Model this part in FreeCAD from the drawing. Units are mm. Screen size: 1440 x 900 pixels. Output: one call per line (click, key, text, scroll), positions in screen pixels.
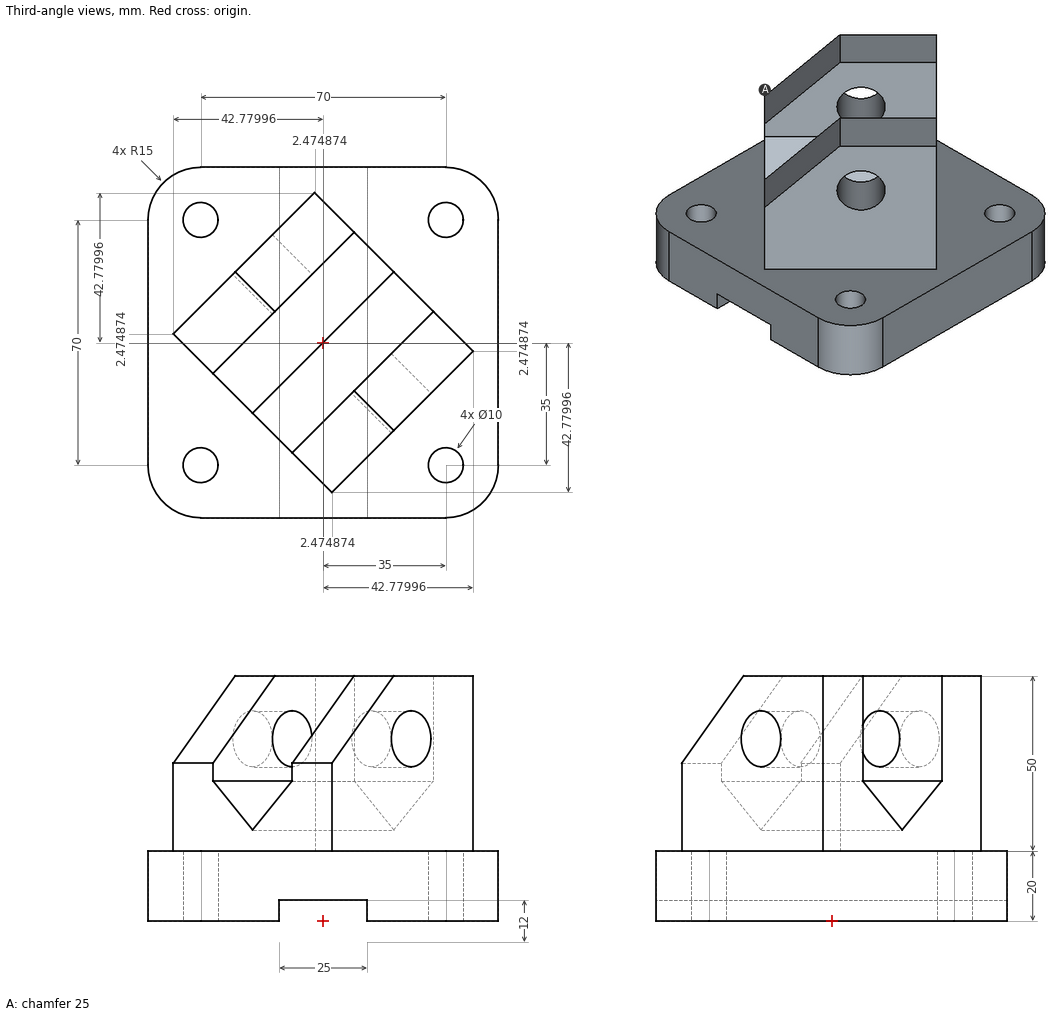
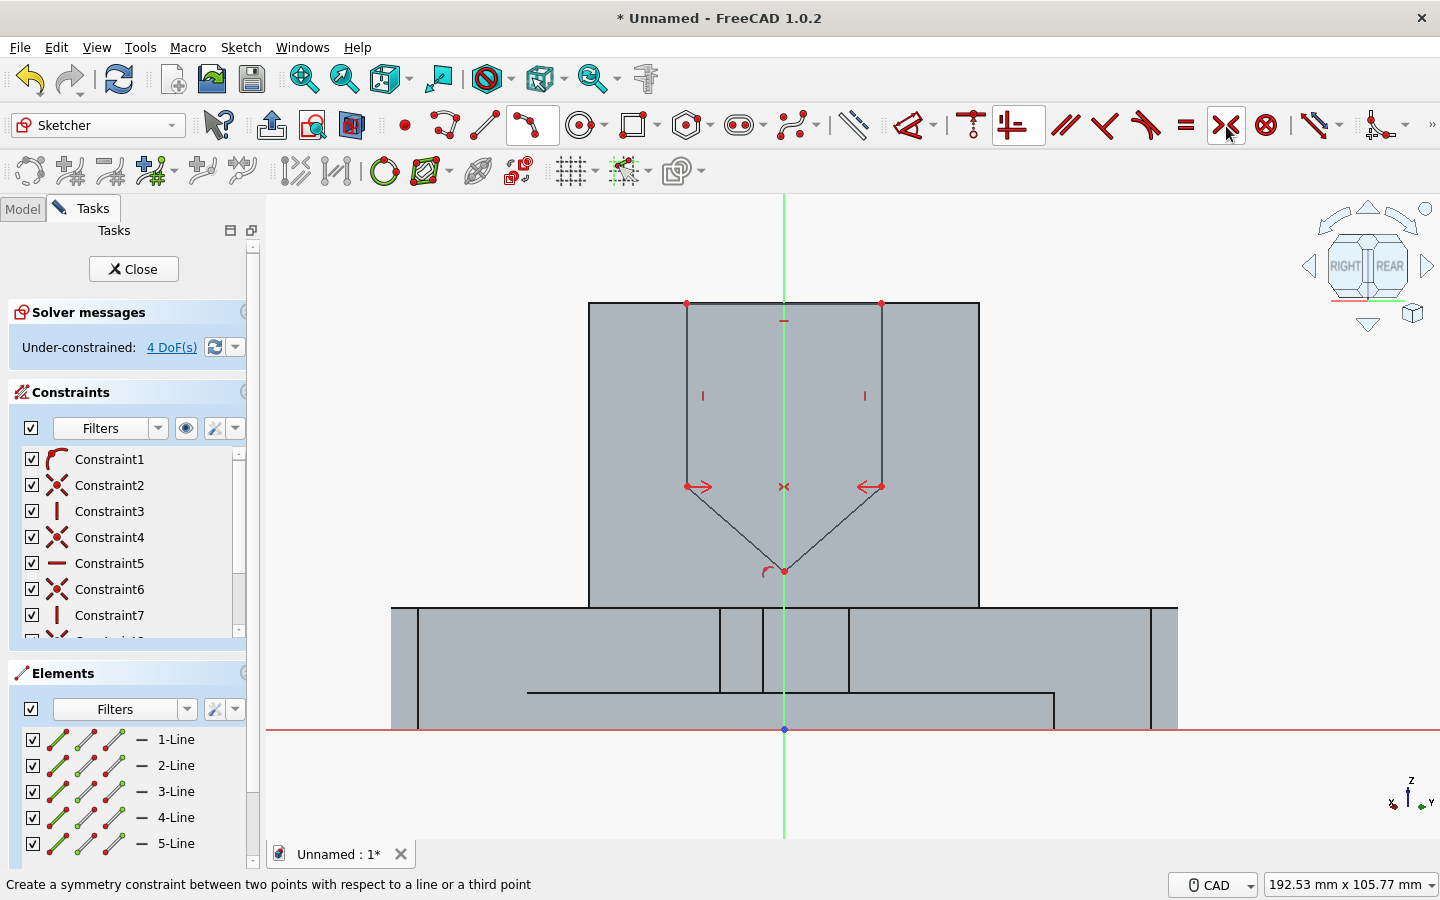
key(d)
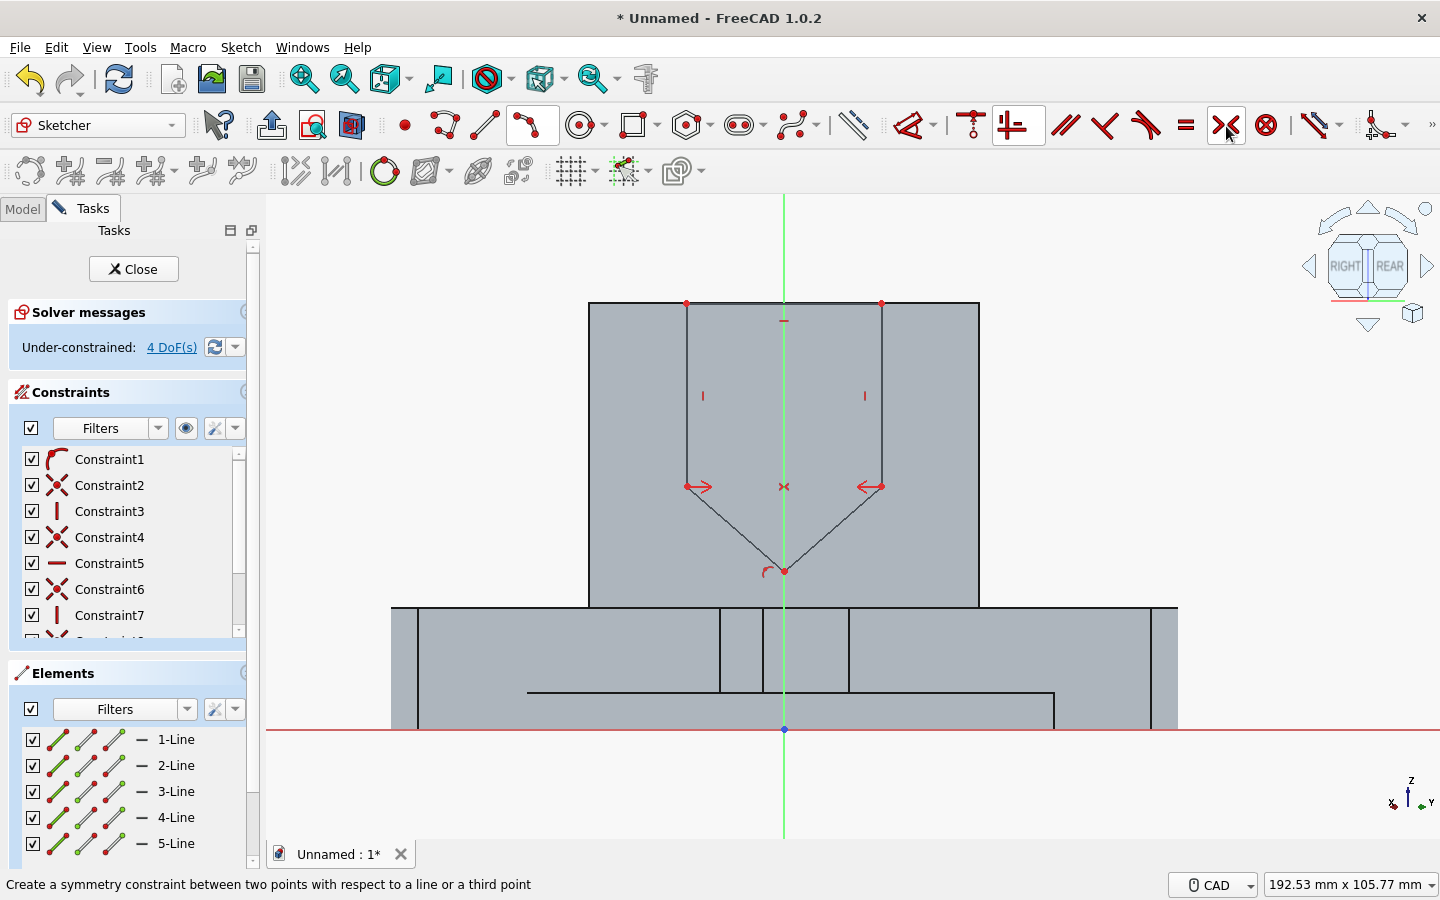
click(882, 432)
click(916, 396)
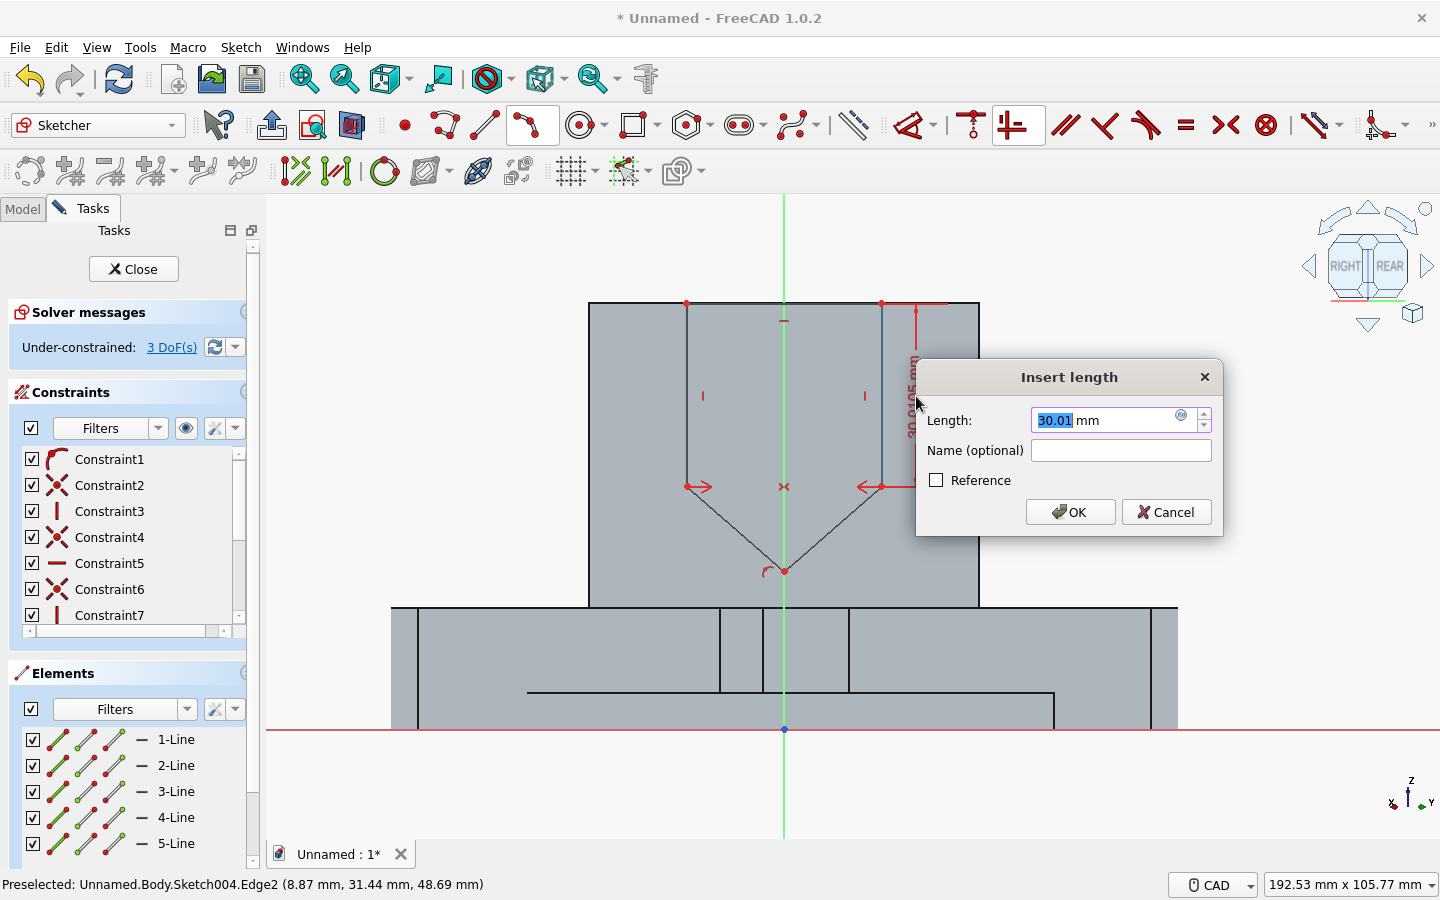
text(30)
key(Return)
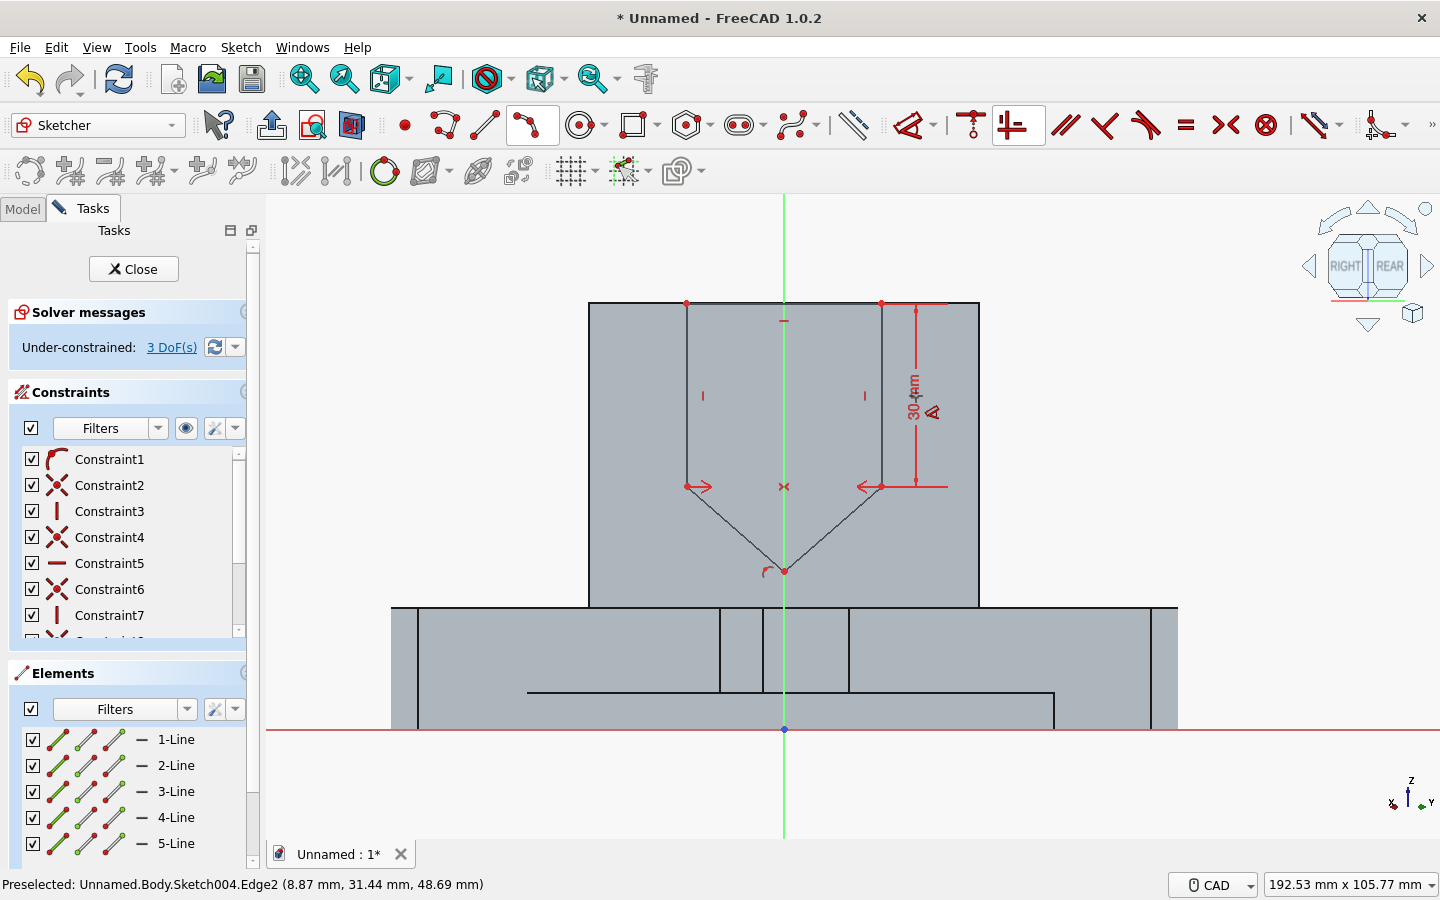
click(823, 304)
click(740, 270)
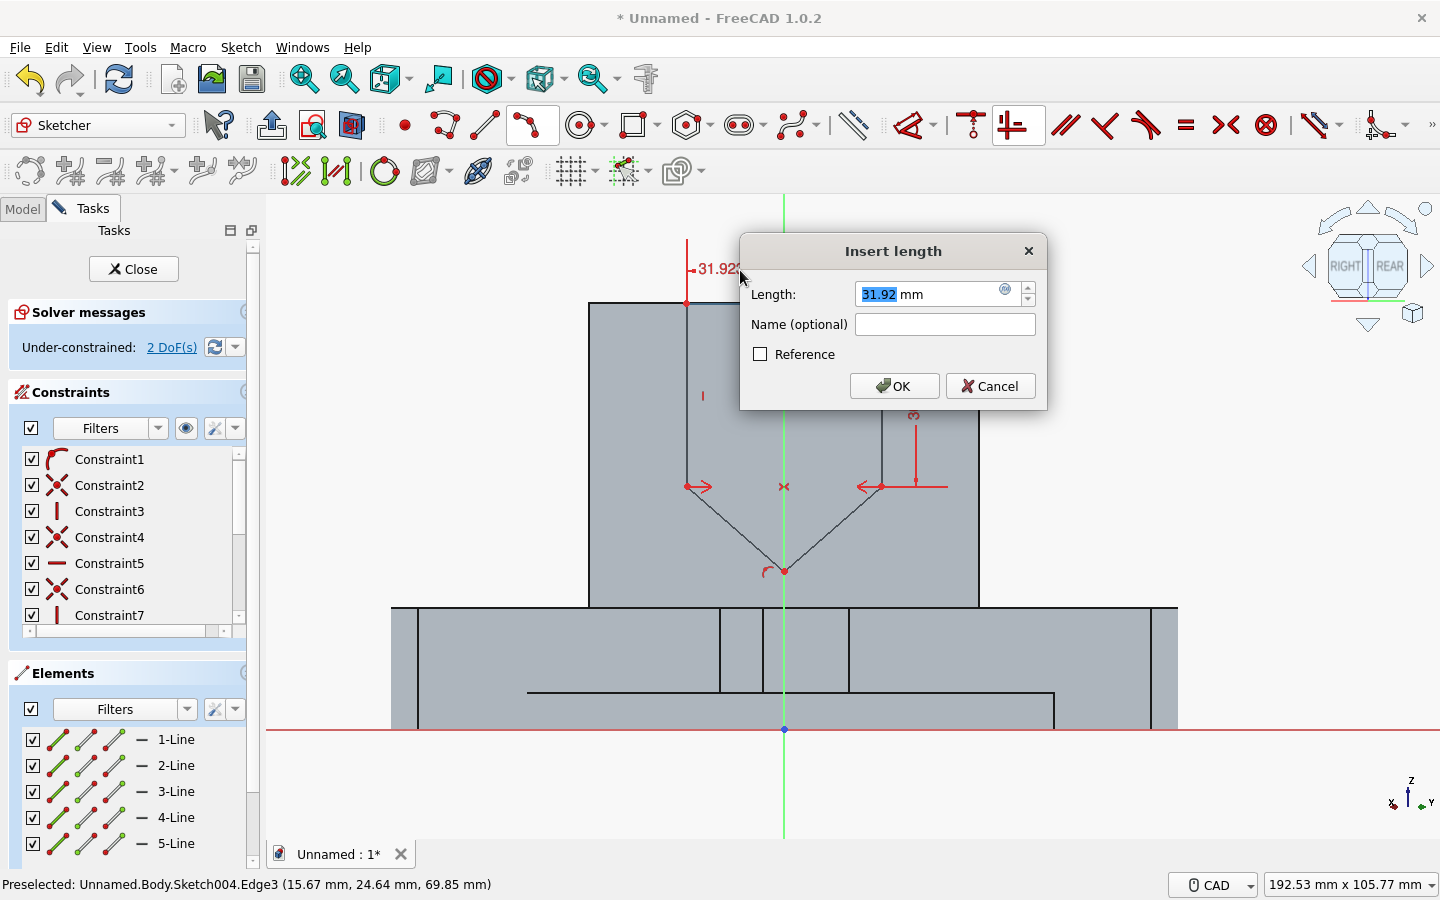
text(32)
key(Return)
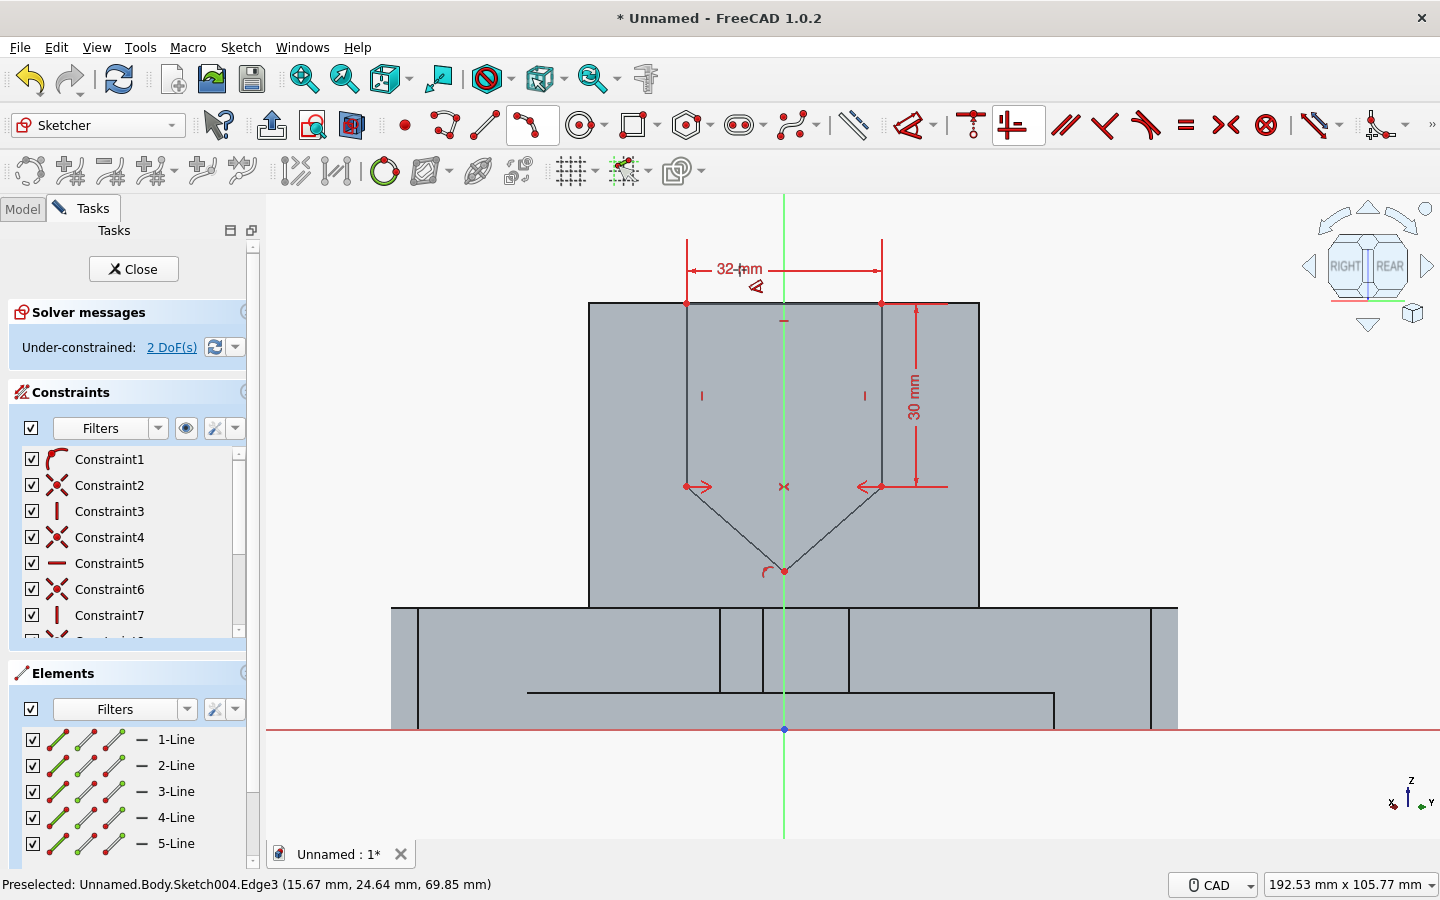
click(784, 572)
click(818, 651)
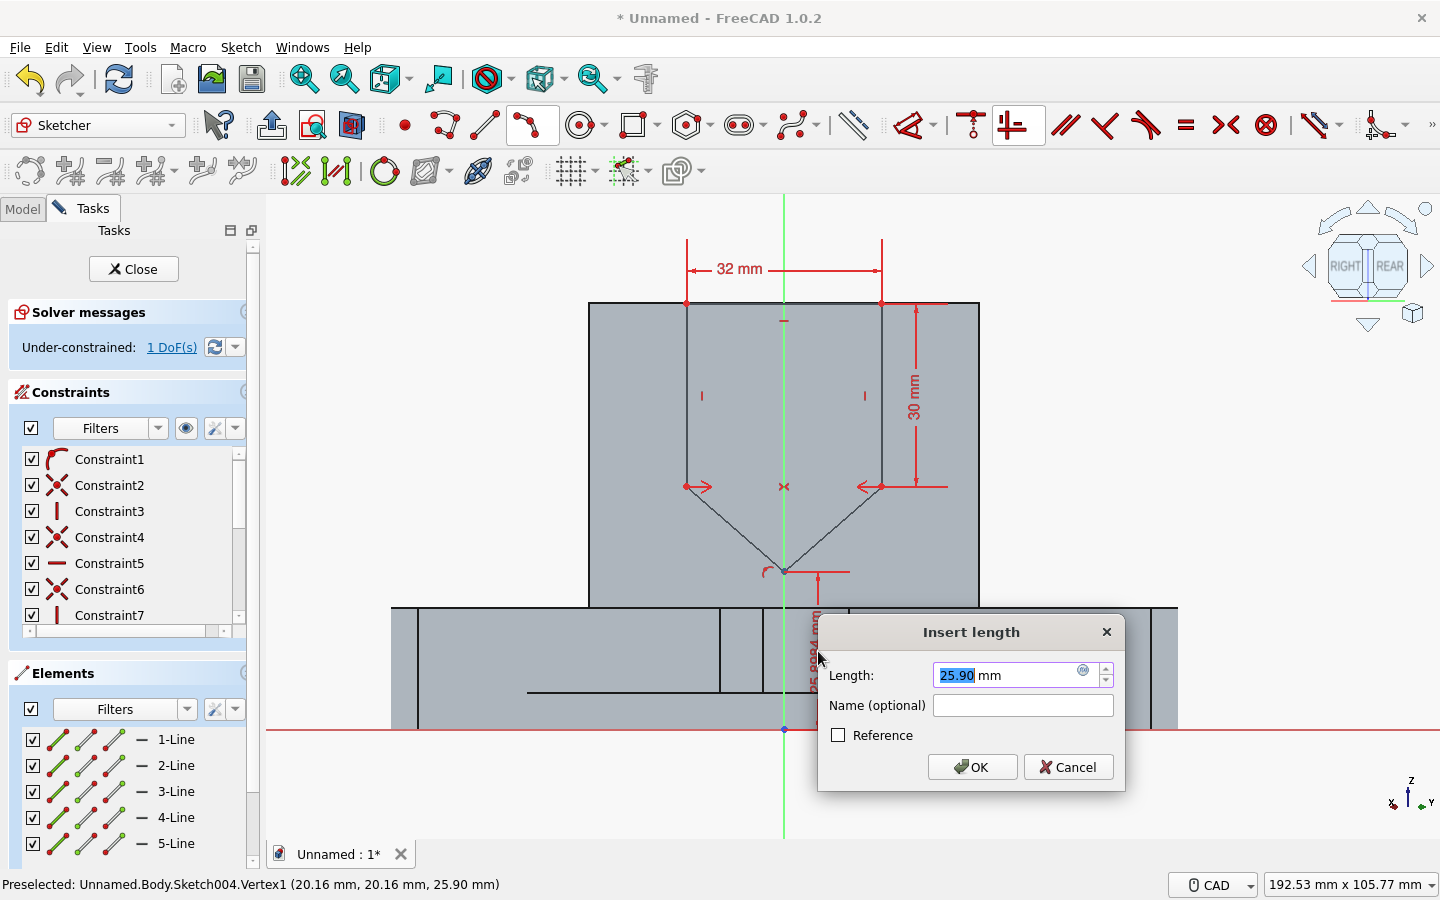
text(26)
key(Return)